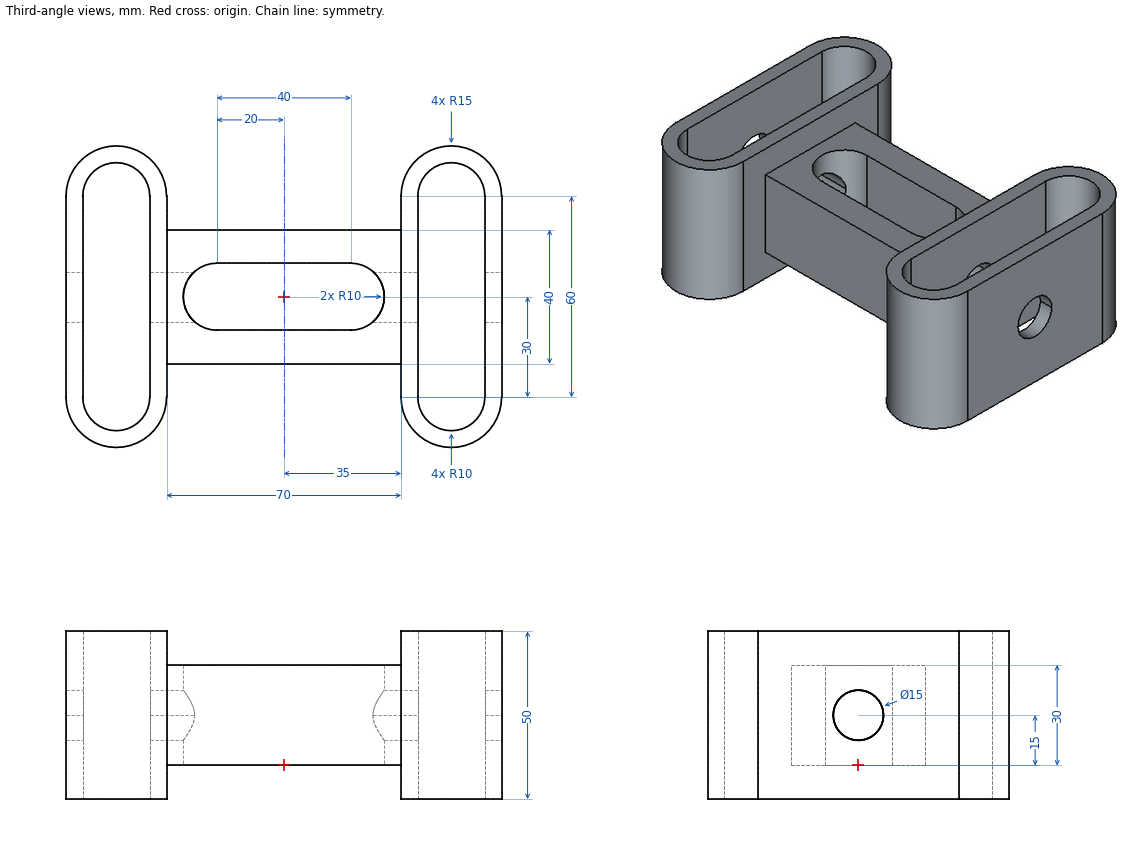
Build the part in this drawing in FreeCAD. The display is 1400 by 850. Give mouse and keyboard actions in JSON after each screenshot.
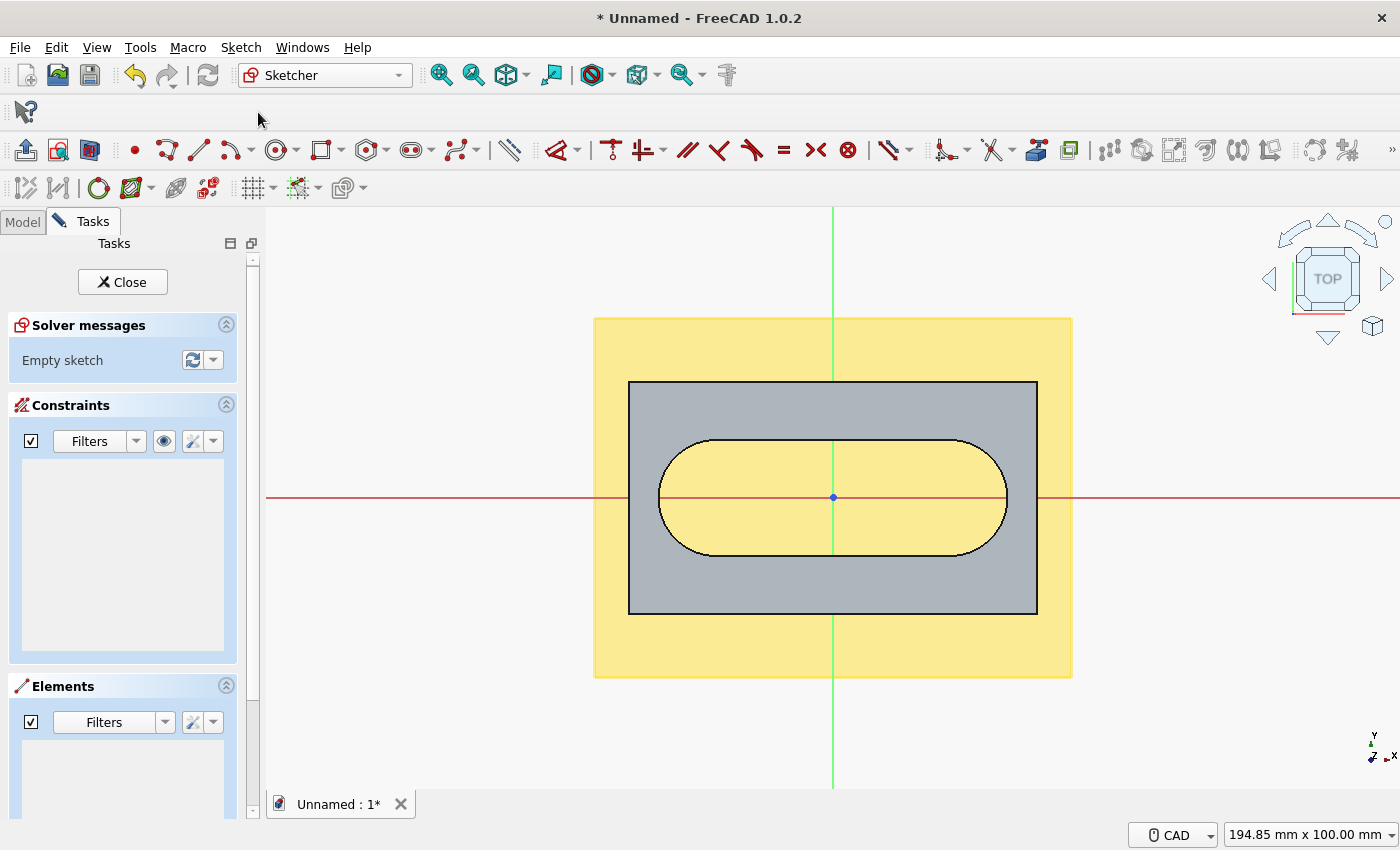
{"action": "key", "text": "q s"}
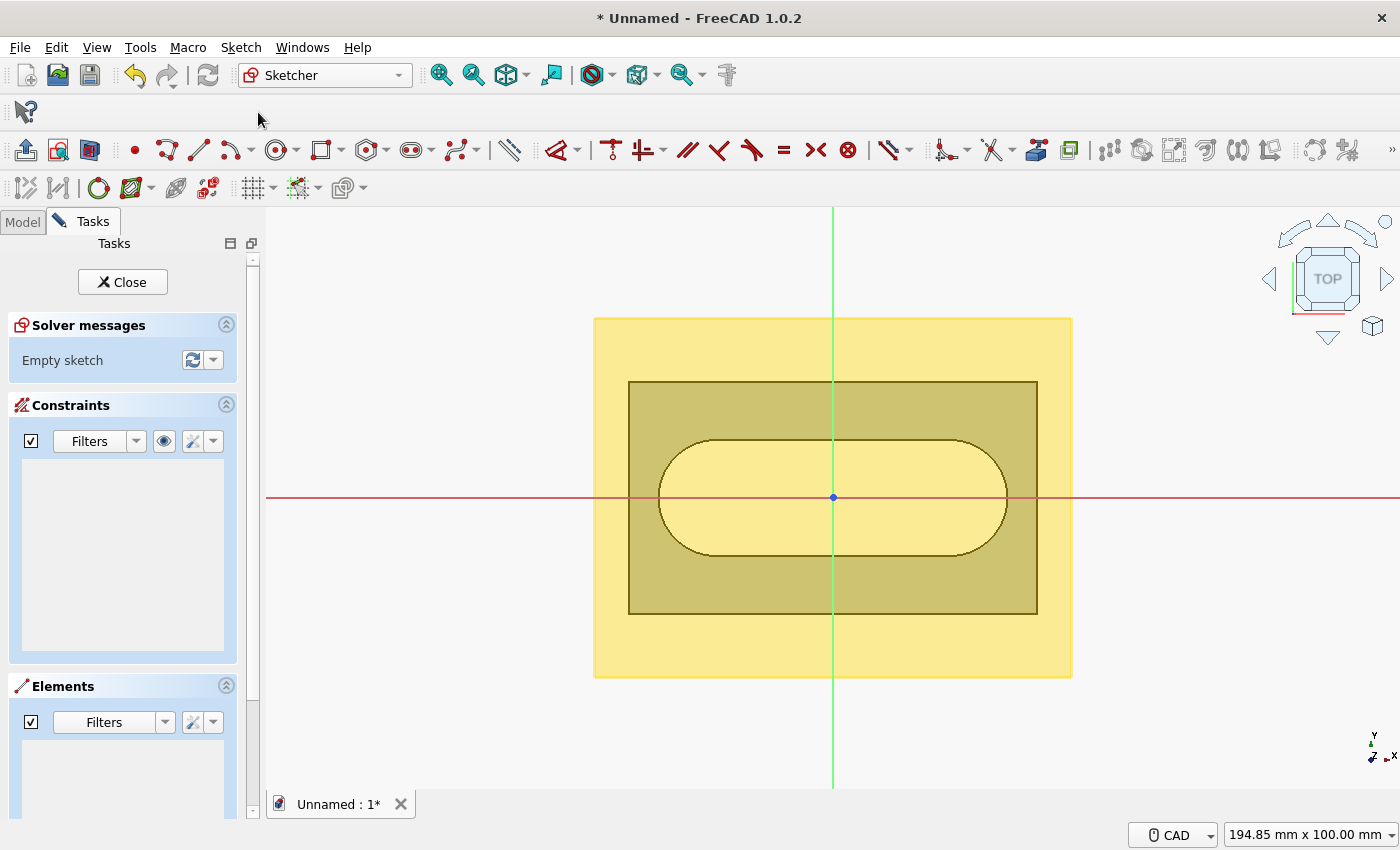
{"action": "scroll", "coordinate": [625, 498], "scroll_direction": "down", "scroll_amount": 2}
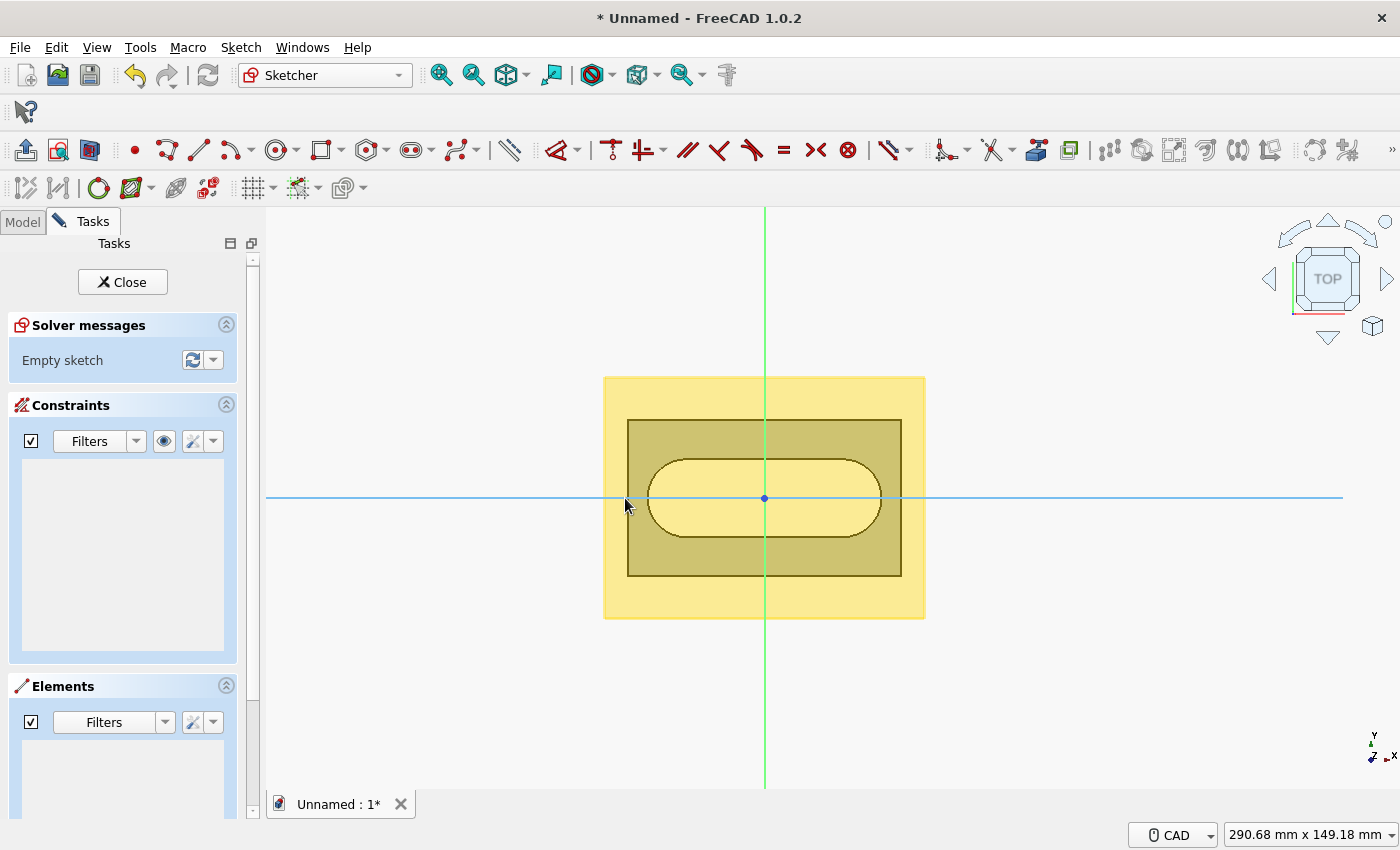
{"action": "key", "text": "g s"}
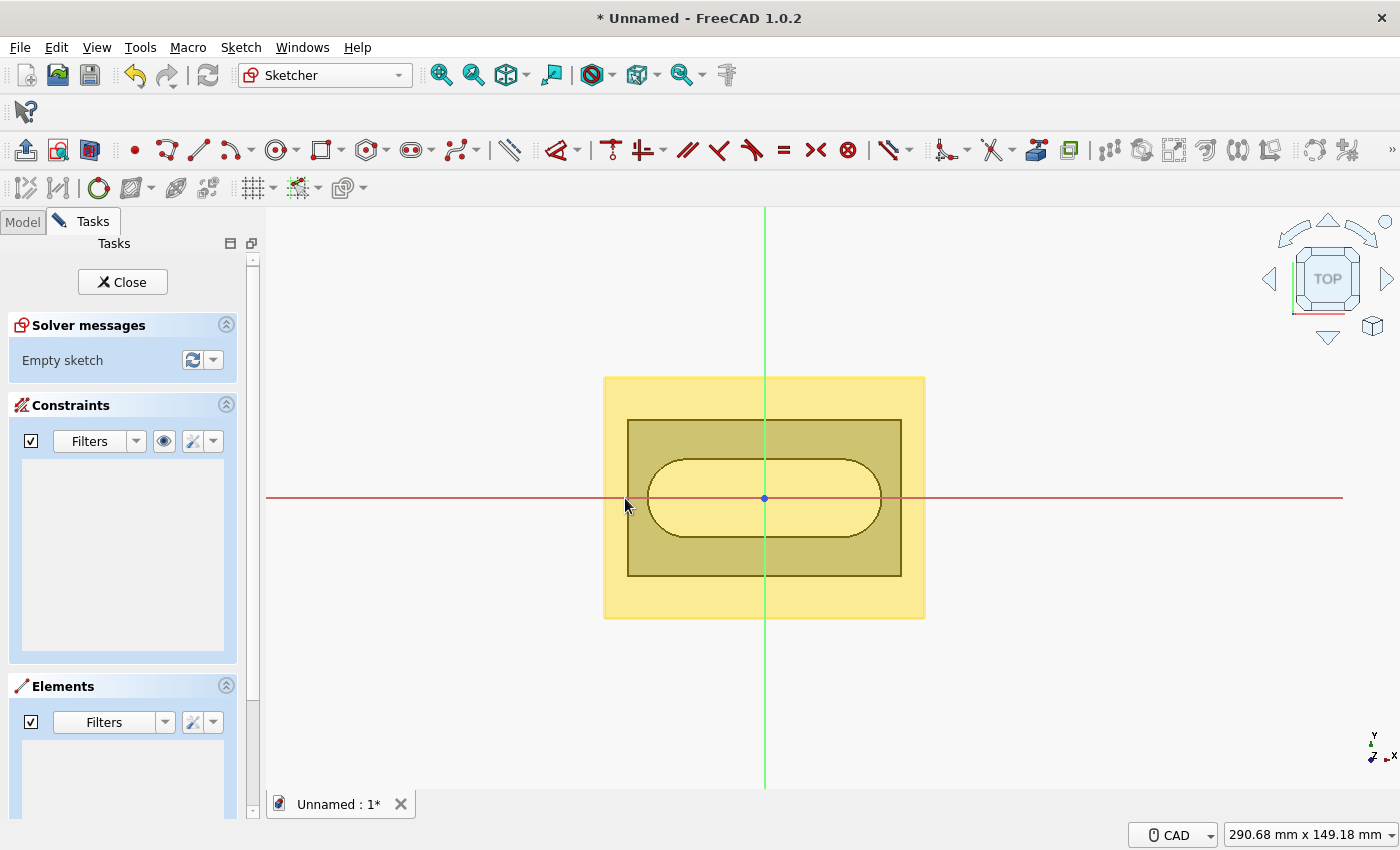
{"action": "left_click", "coordinate": [960, 615]}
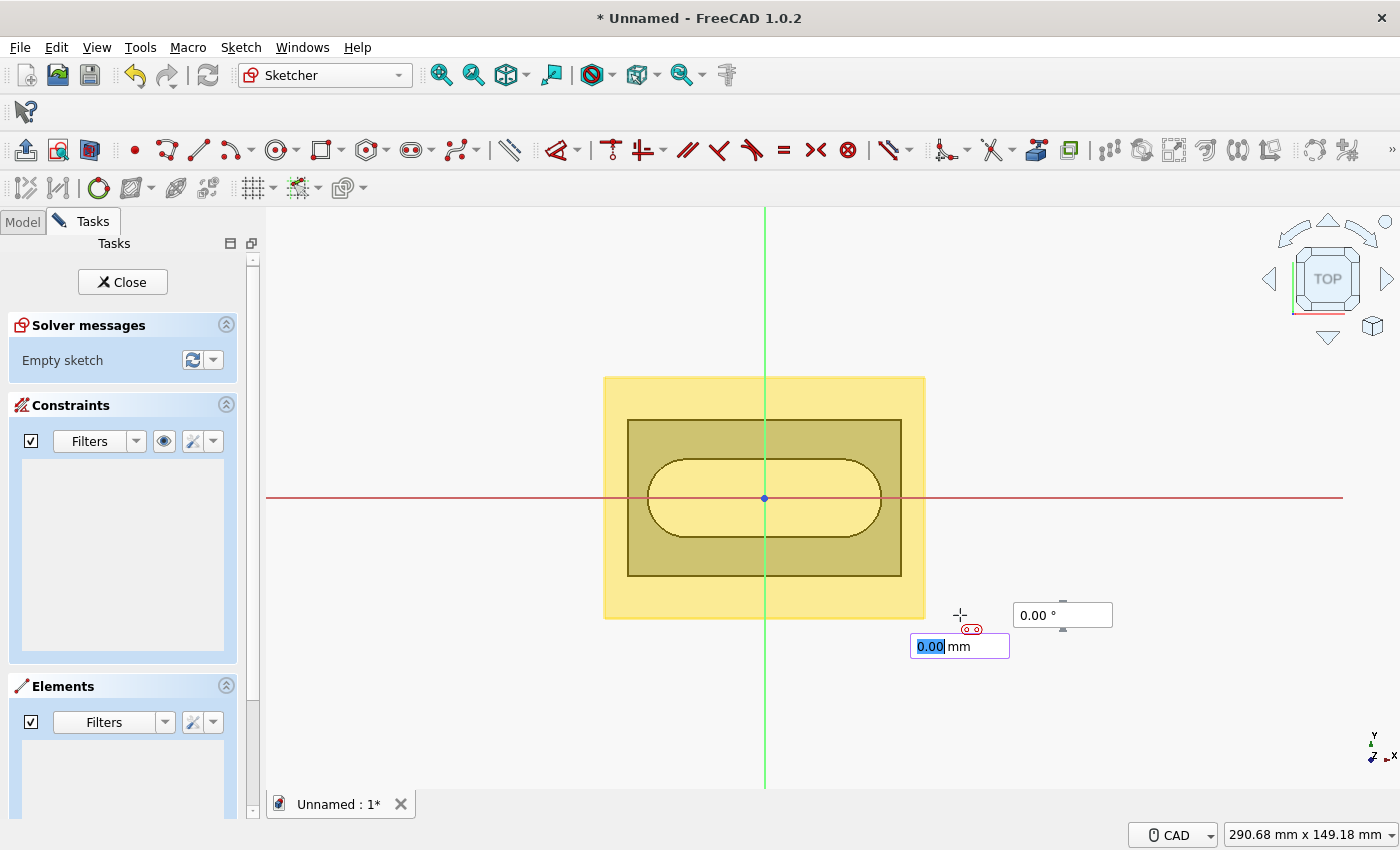
{"action": "left_click", "coordinate": [960, 381]}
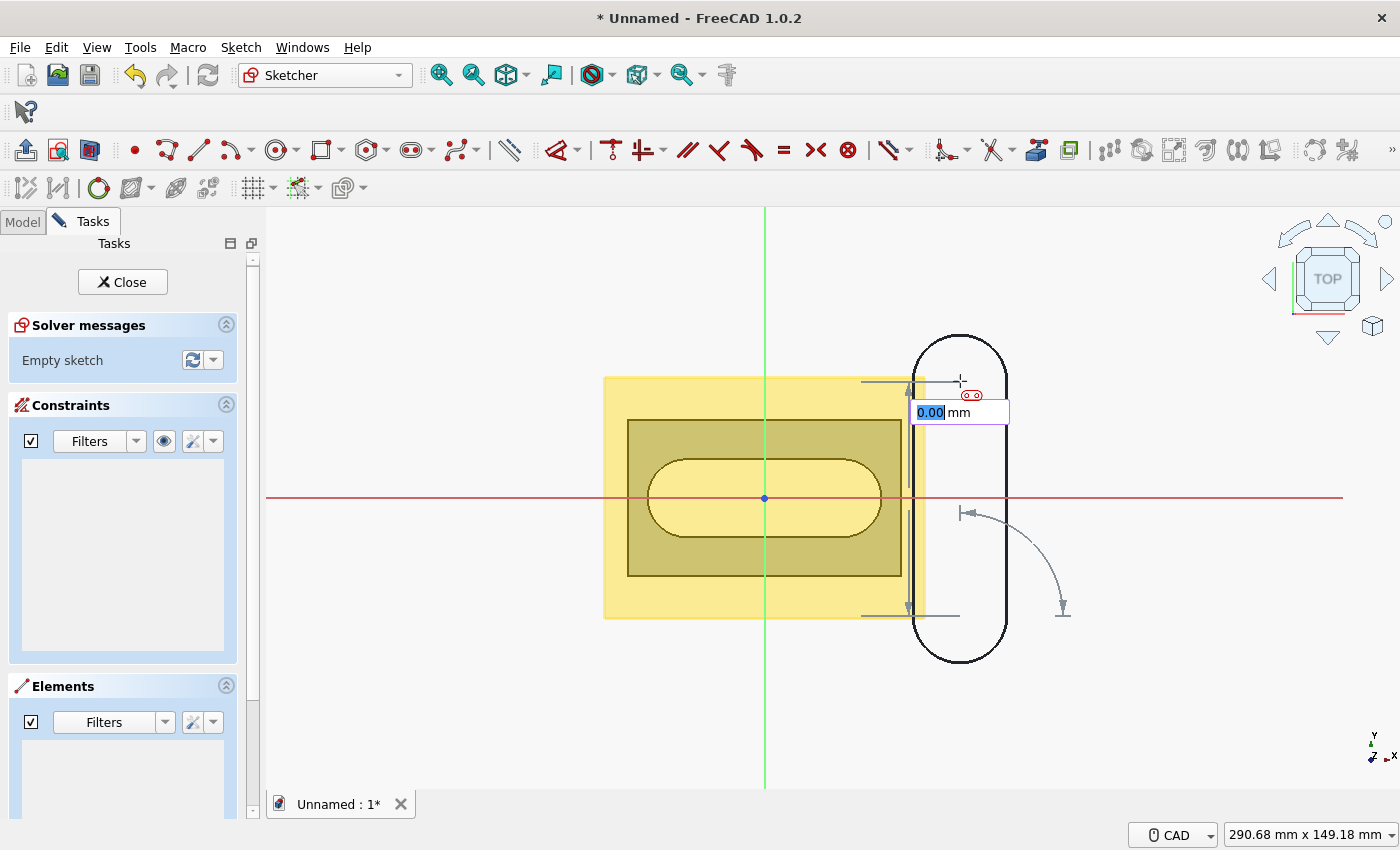
{"action": "left_click", "coordinate": [1018, 533]}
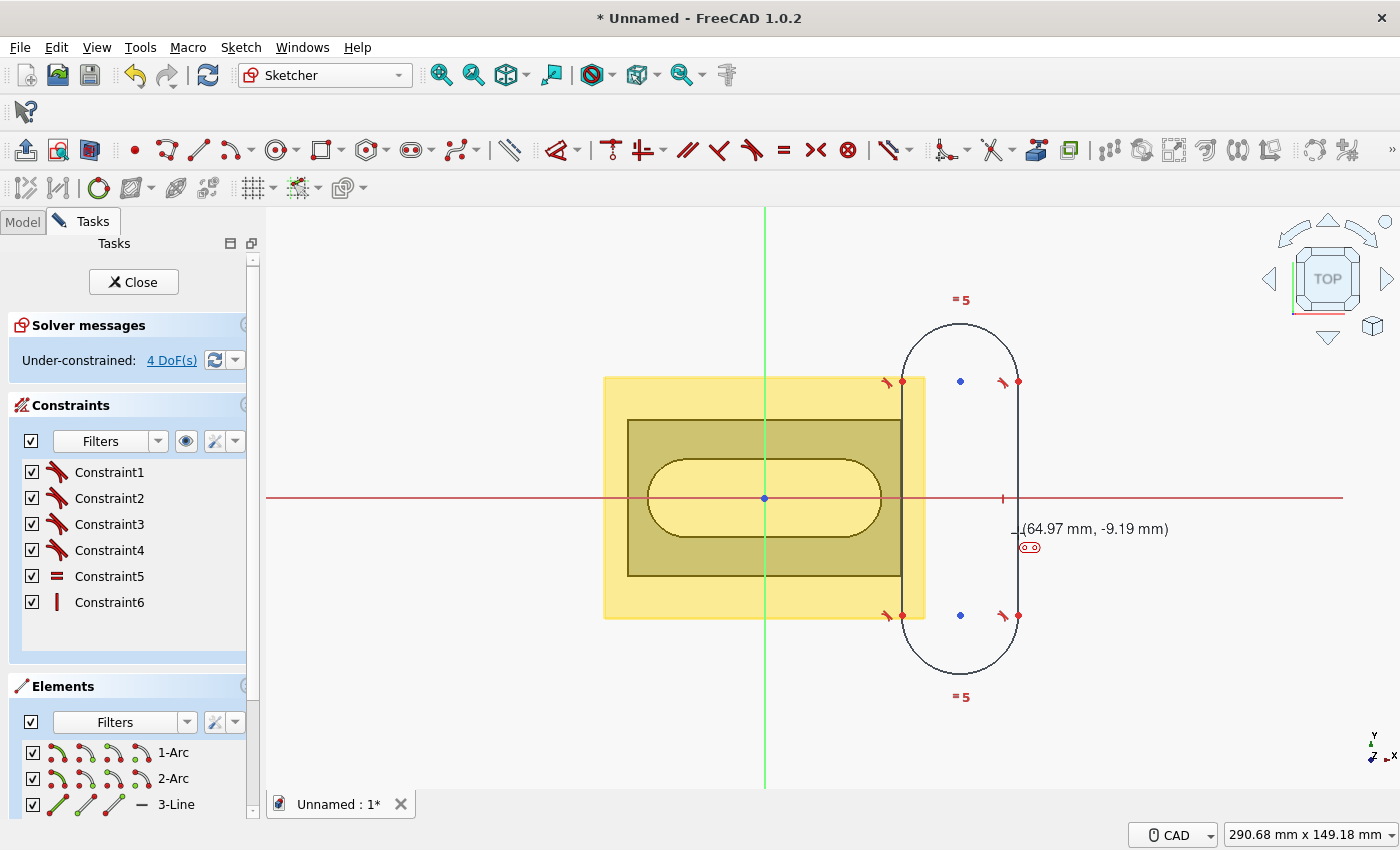
{"action": "left_click", "coordinate": [569, 615]}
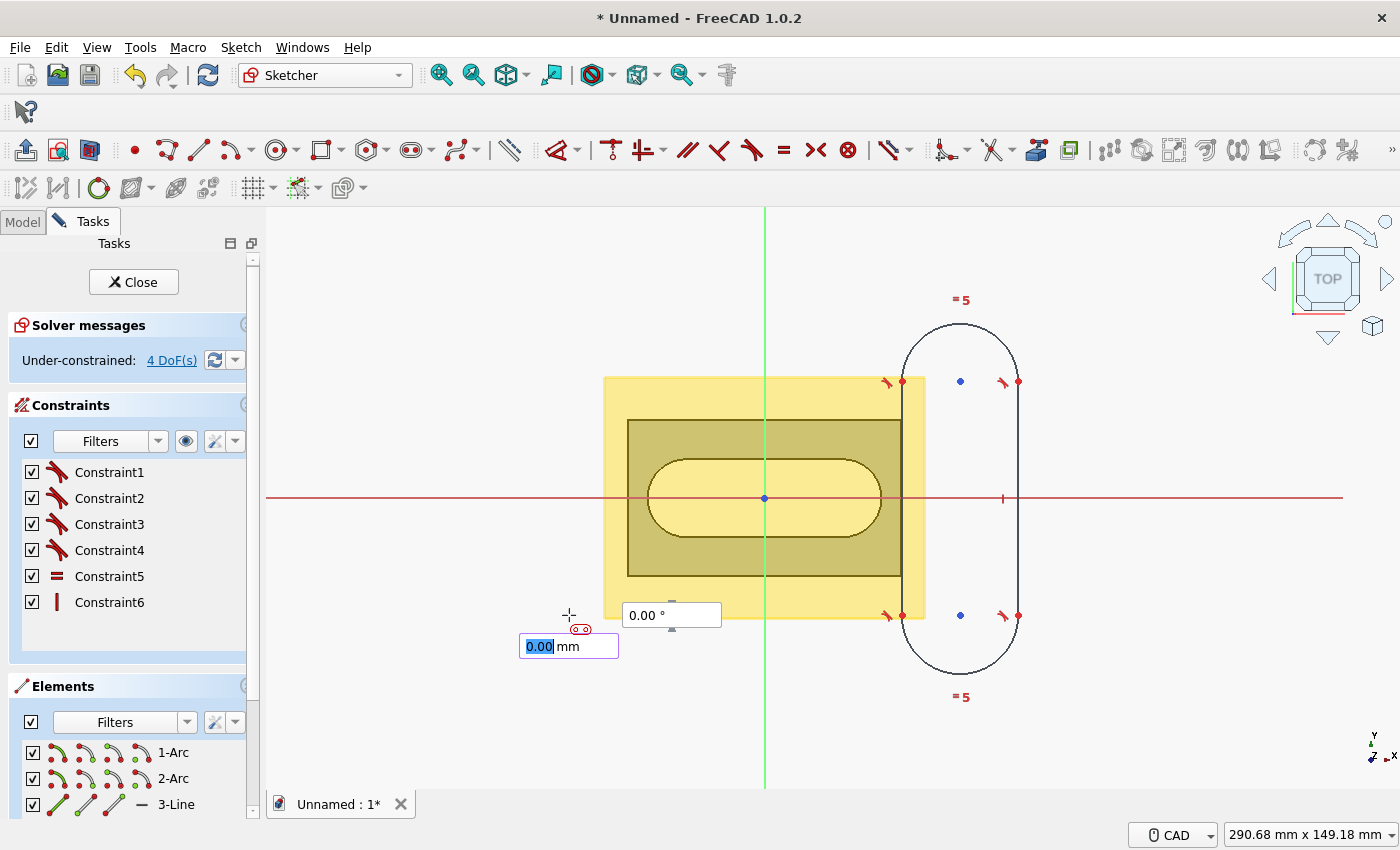
{"action": "left_click", "coordinate": [569, 381]}